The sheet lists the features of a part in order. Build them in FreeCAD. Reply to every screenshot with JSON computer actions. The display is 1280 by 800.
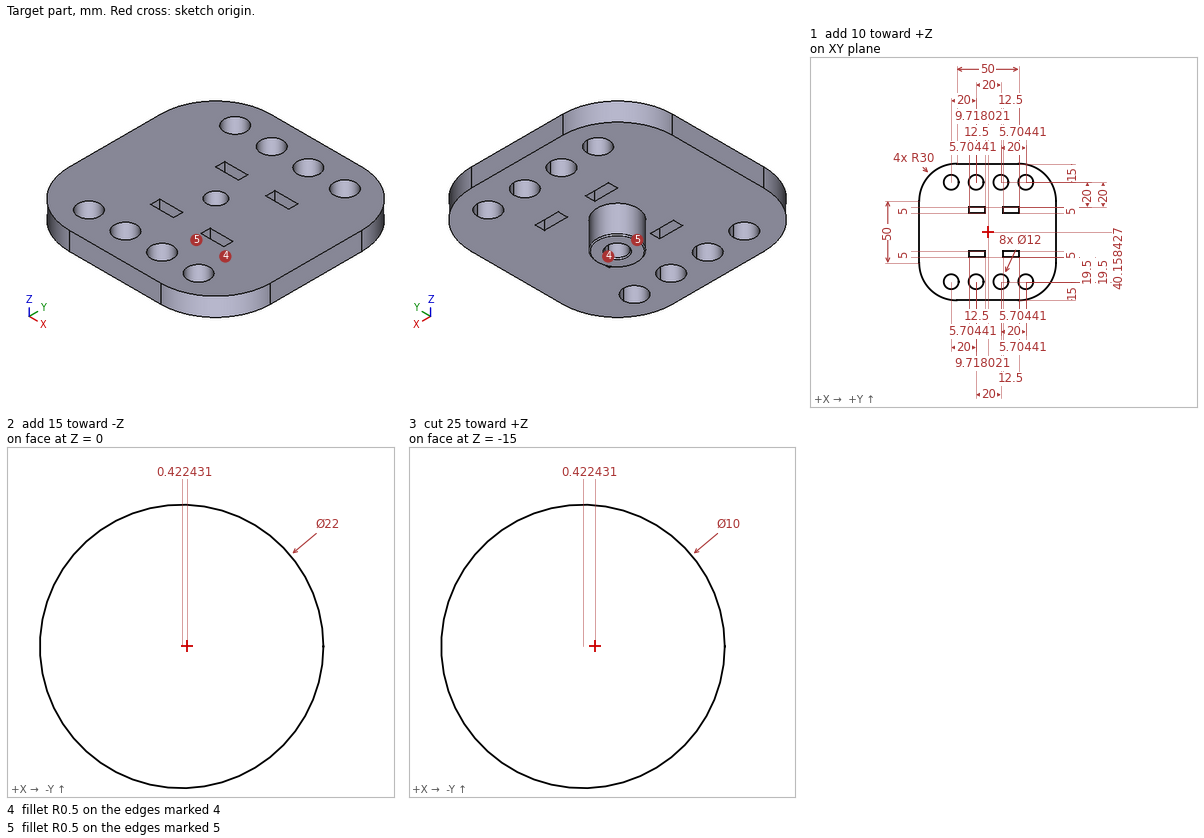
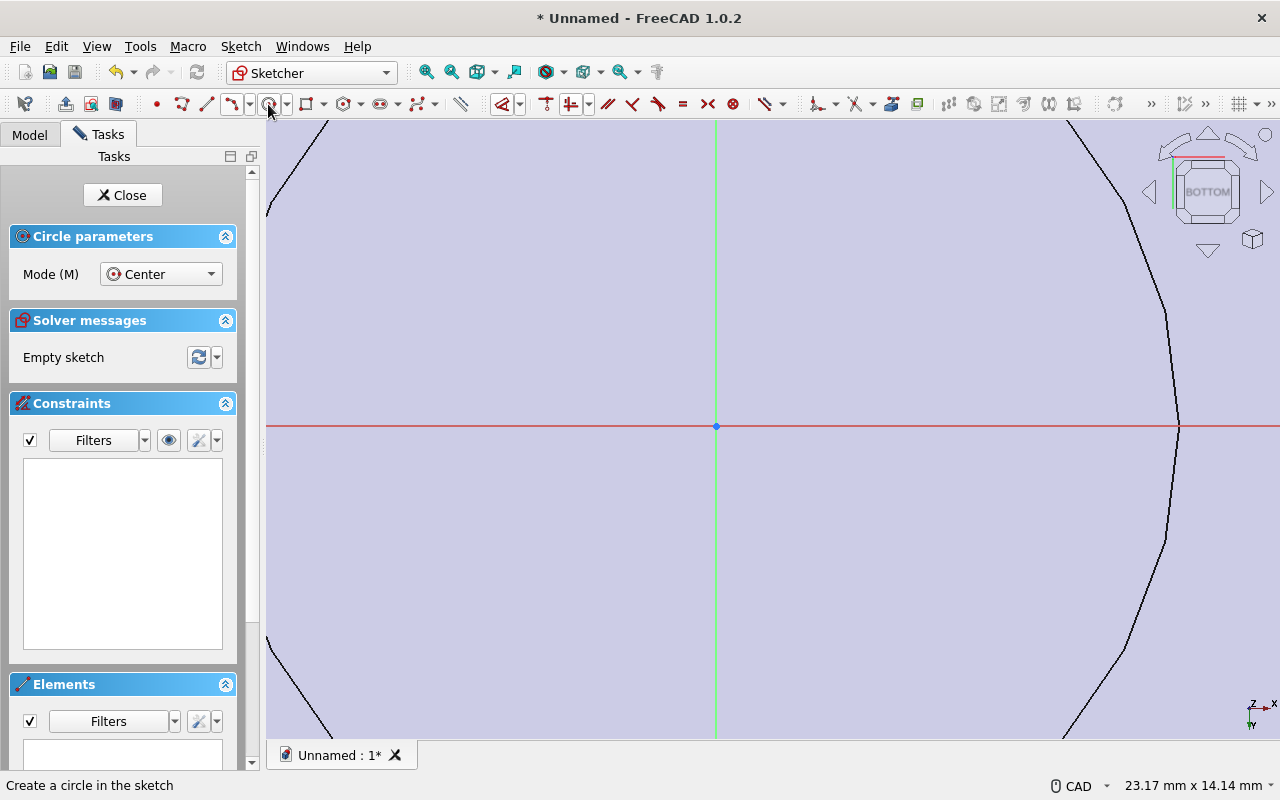
{"action": "left_click", "coordinate": [698, 426]}
{"action": "mouse_move", "coordinate": [853, 272]}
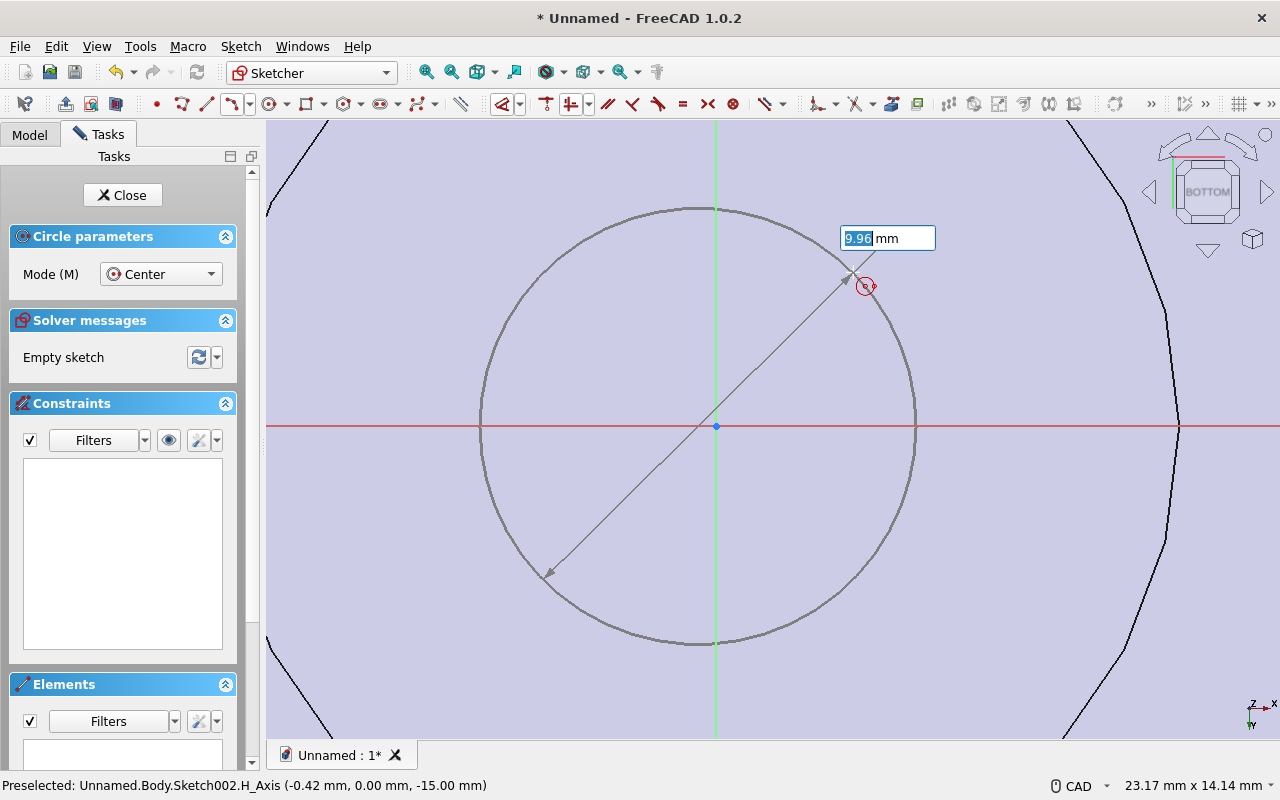
{"action": "type", "text": "10"}
{"action": "key", "text": "Return"}
{"action": "key", "text": "Escape"}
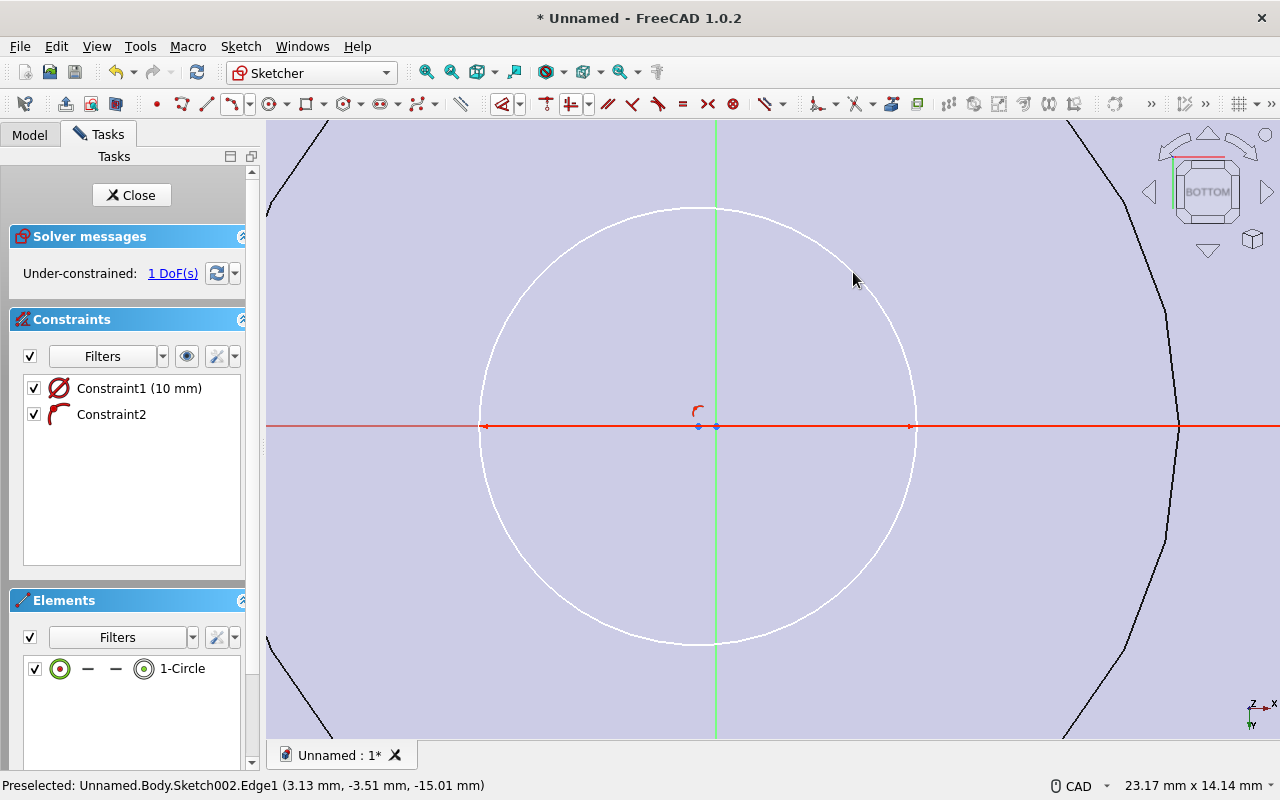
{"action": "scroll", "coordinate": [698, 426], "scroll_direction": "up", "scroll_amount": 4}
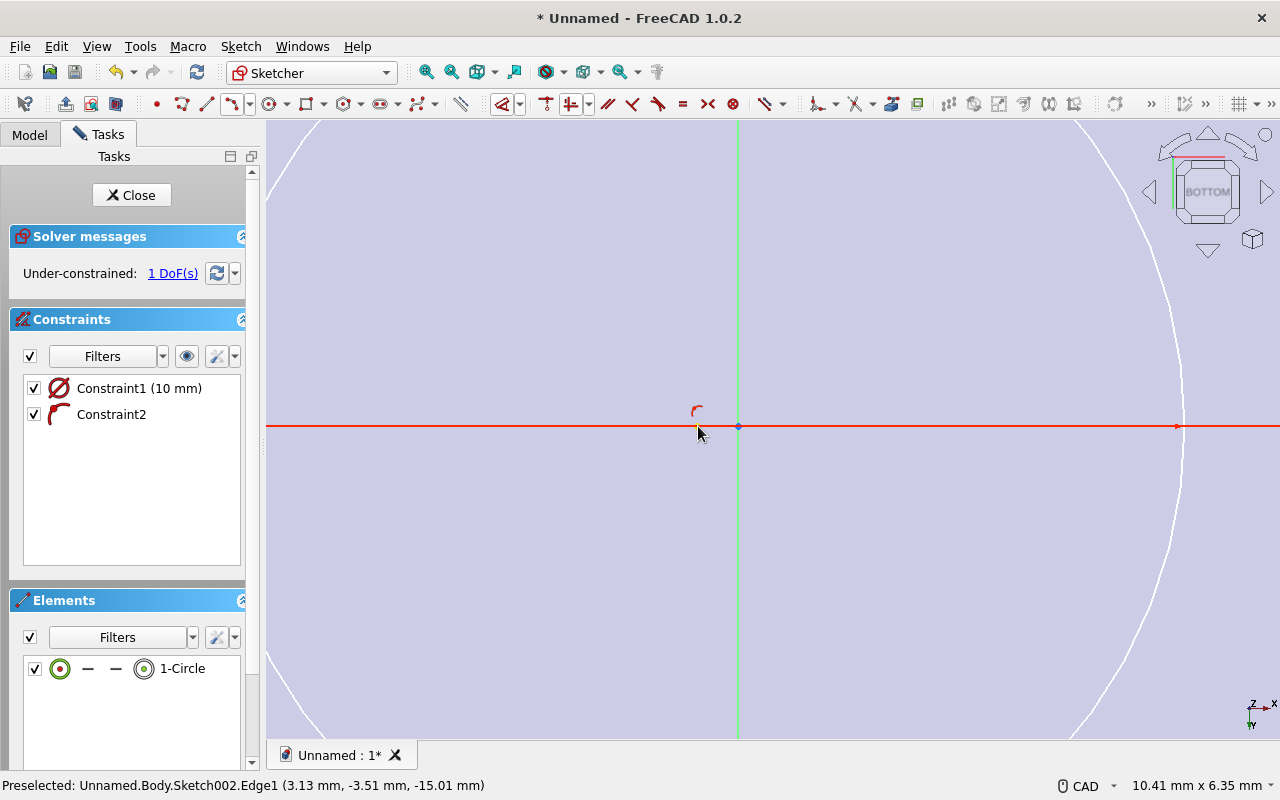
{"action": "left_click", "coordinate": [697, 426]}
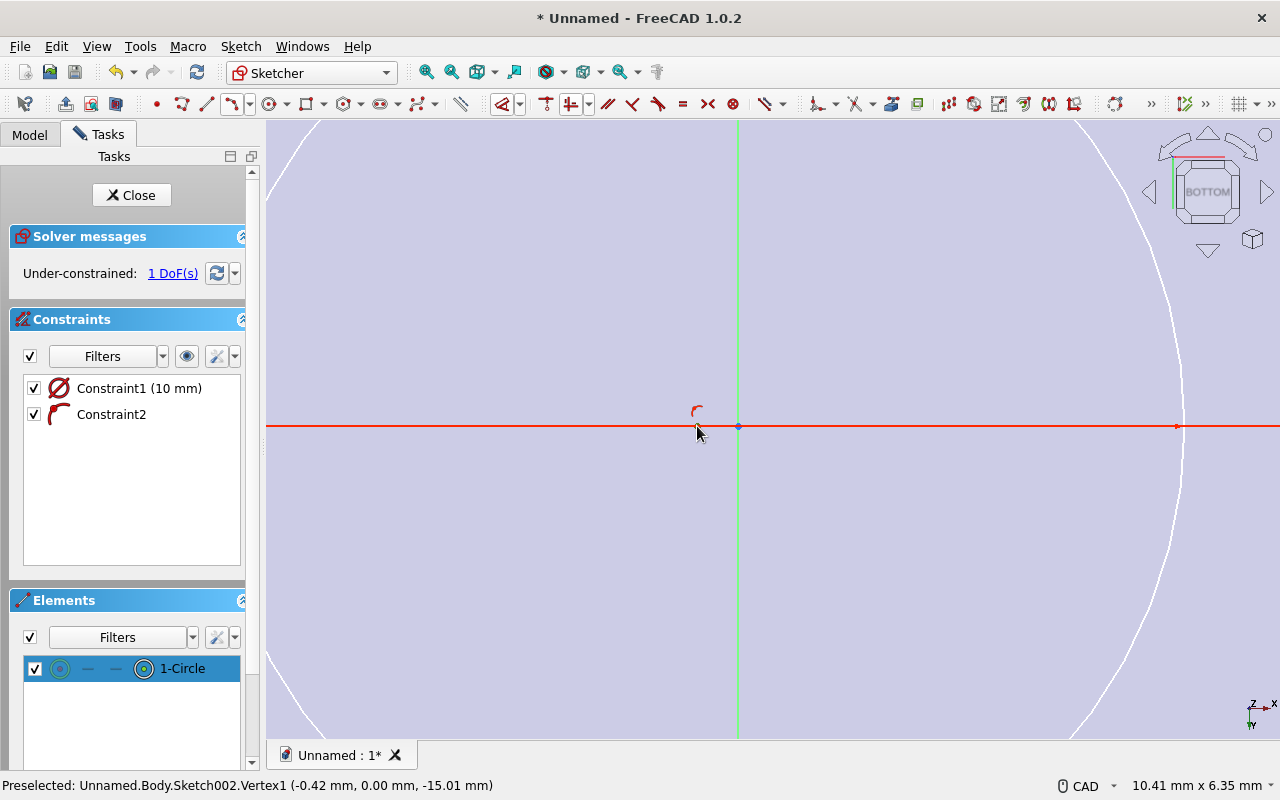
{"action": "key", "text": "l"}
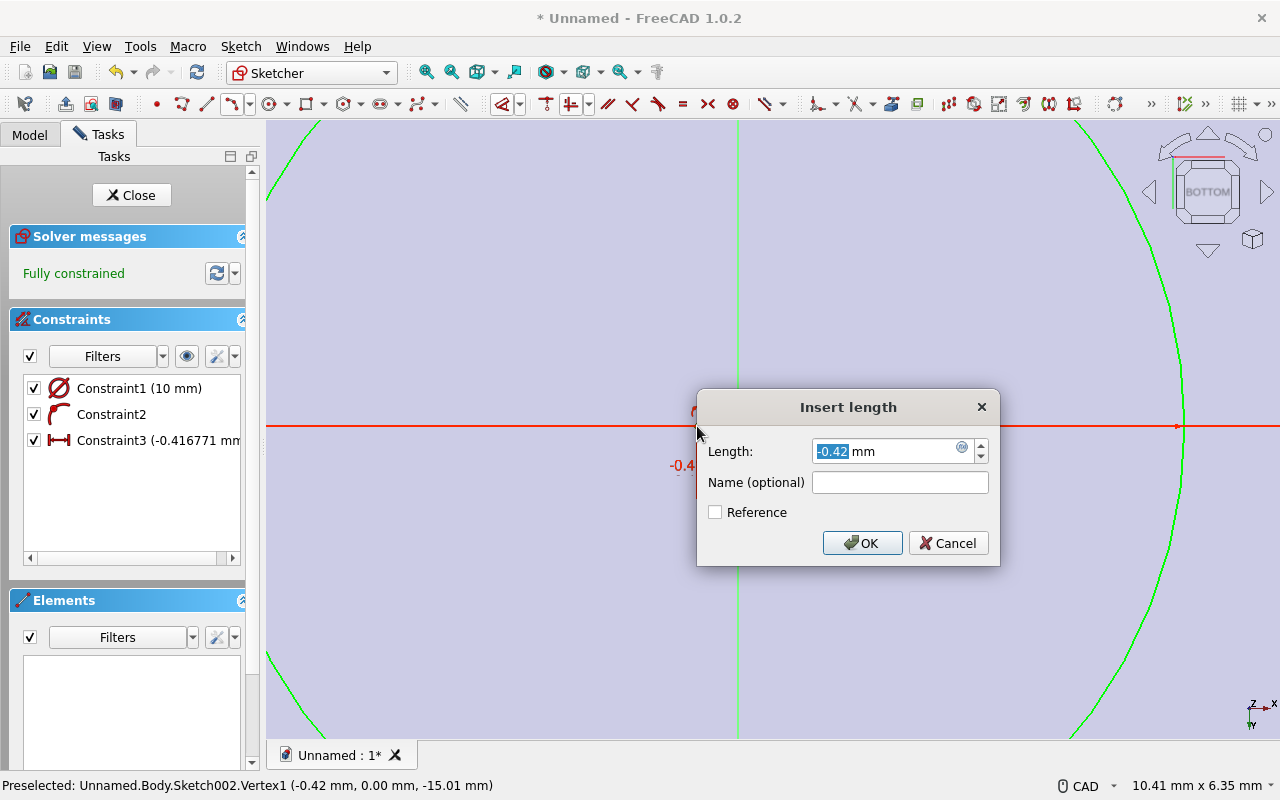
{"action": "type", "text": "-0.422431"}
{"action": "key", "text": "Return"}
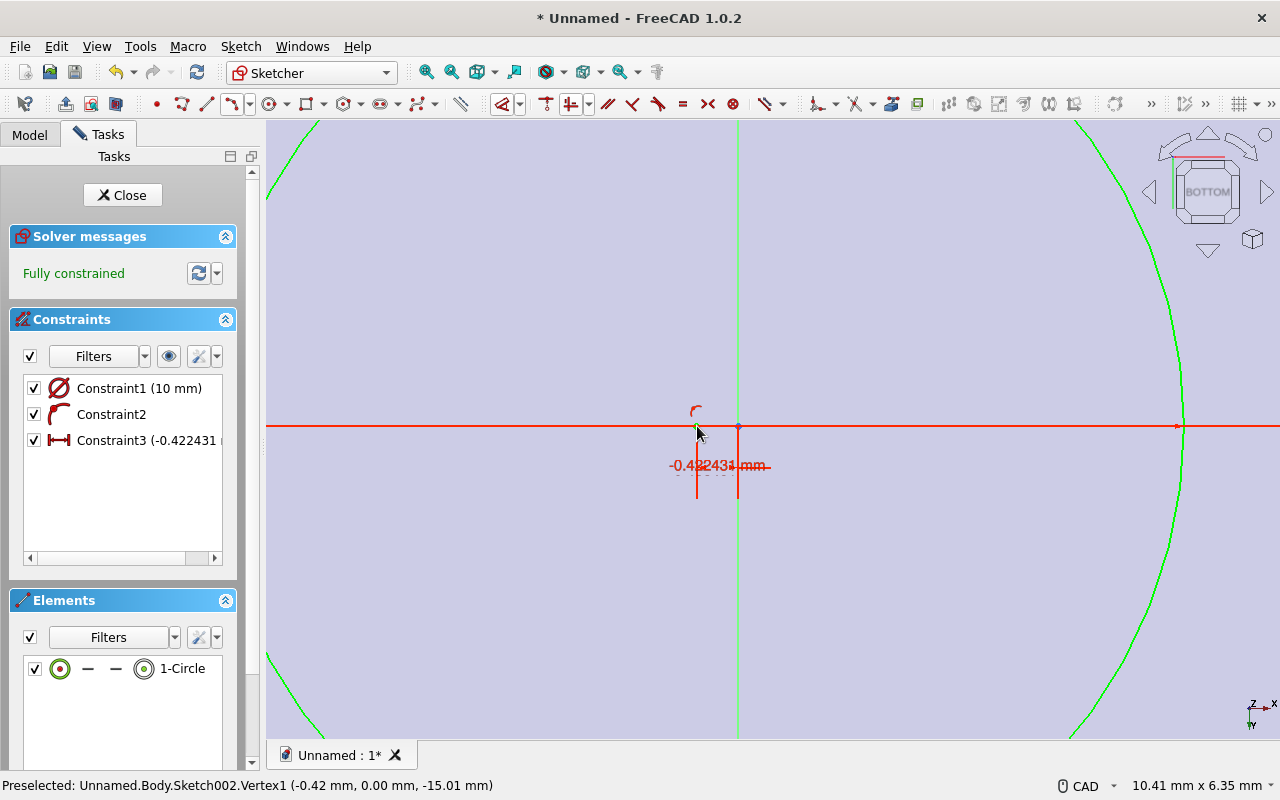
{"action": "left_click", "coordinate": [123, 195]}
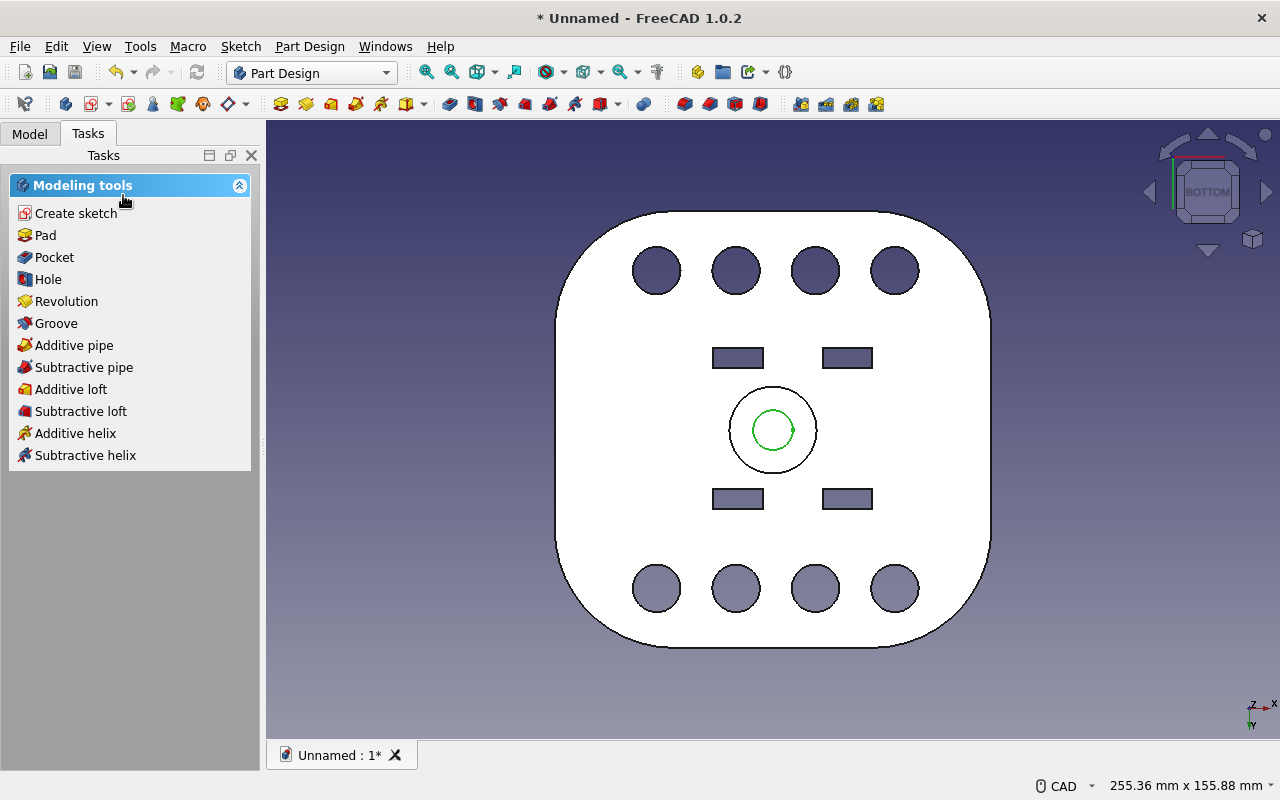
{"action": "left_click", "coordinate": [450, 104]}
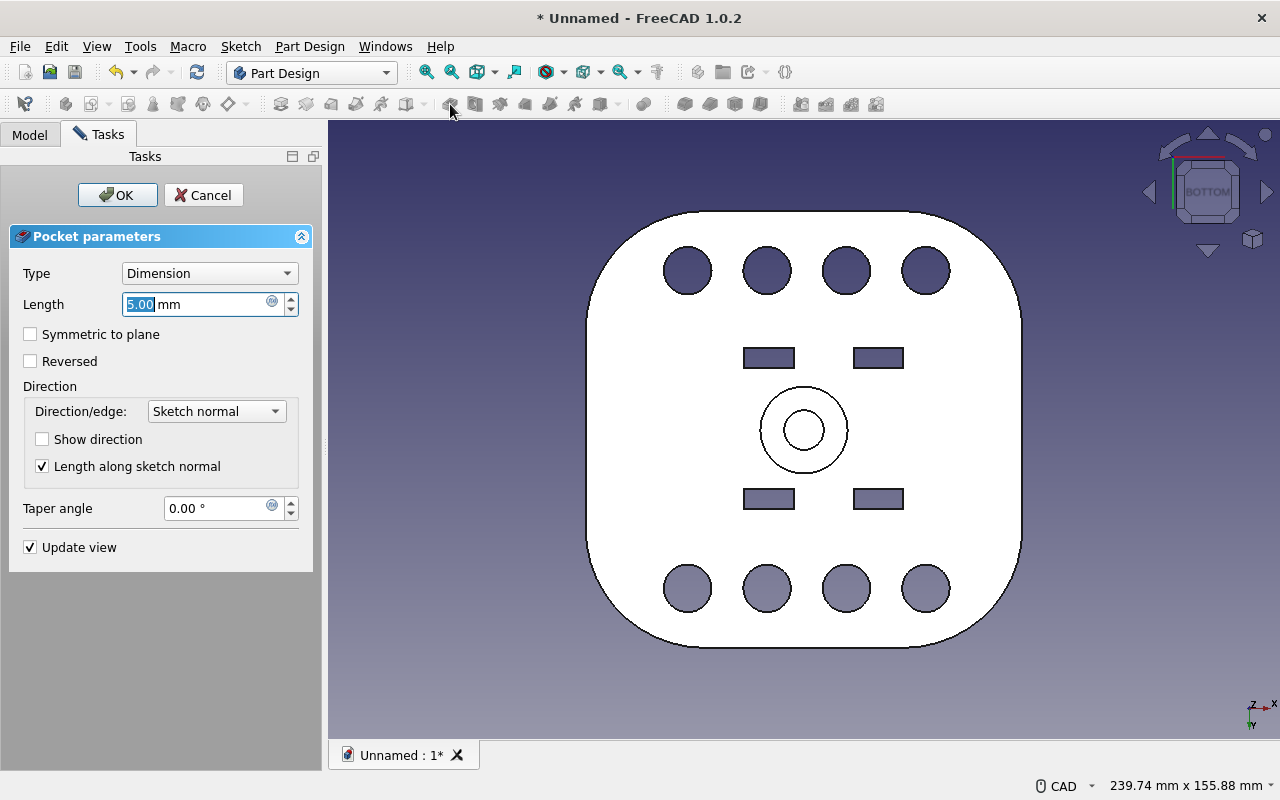
{"action": "type", "text": "25"}
{"action": "key", "text": "Tab"}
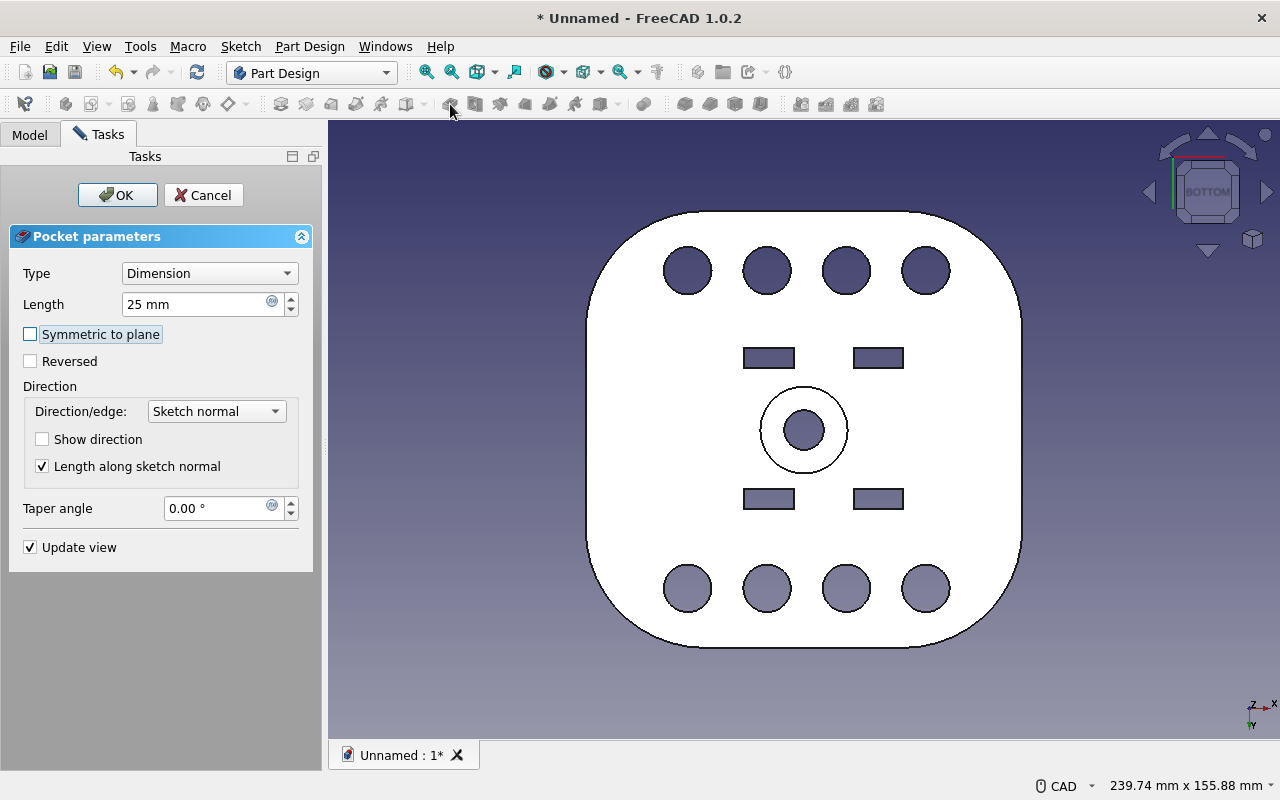
{"action": "left_click", "coordinate": [118, 195]}